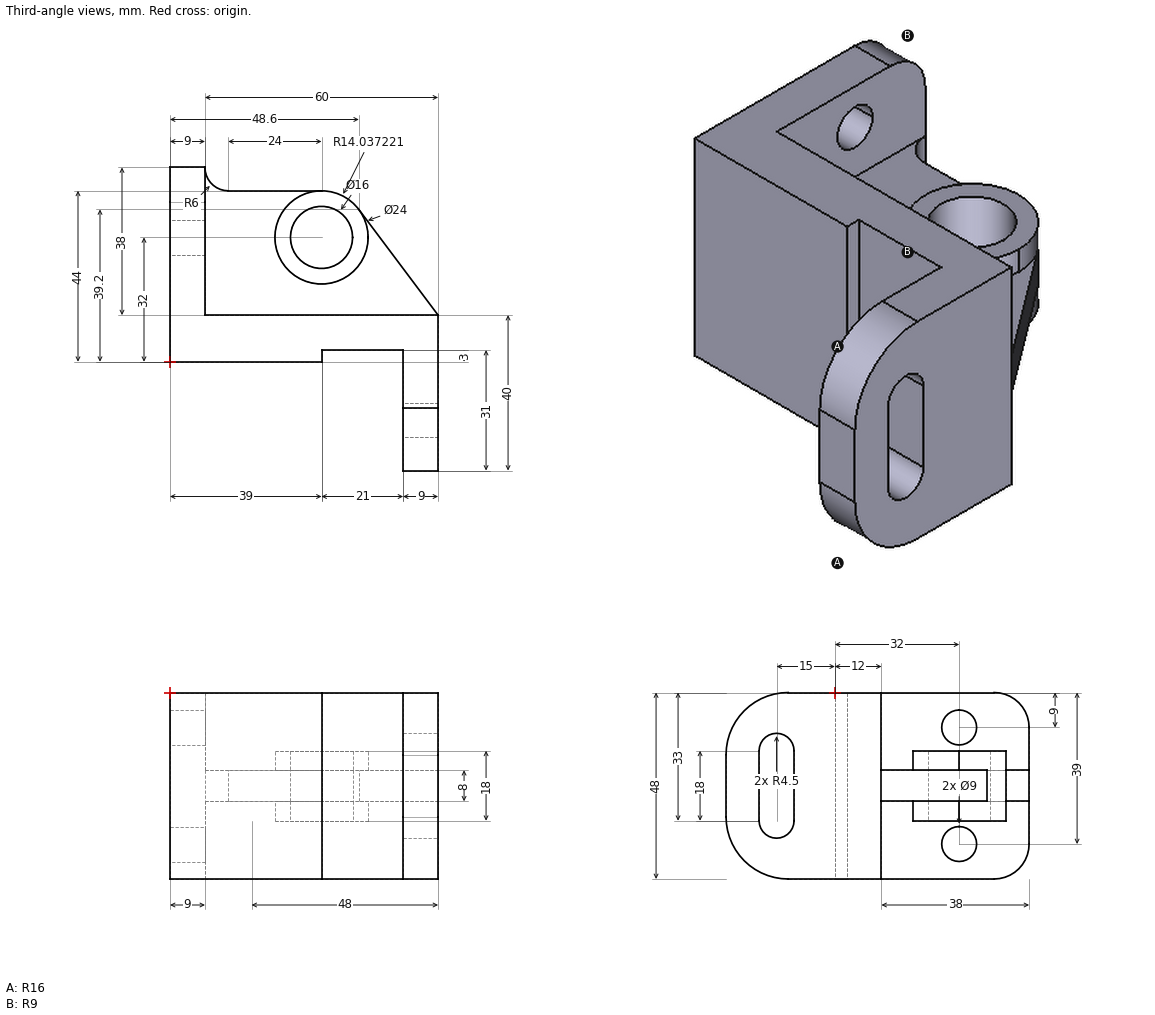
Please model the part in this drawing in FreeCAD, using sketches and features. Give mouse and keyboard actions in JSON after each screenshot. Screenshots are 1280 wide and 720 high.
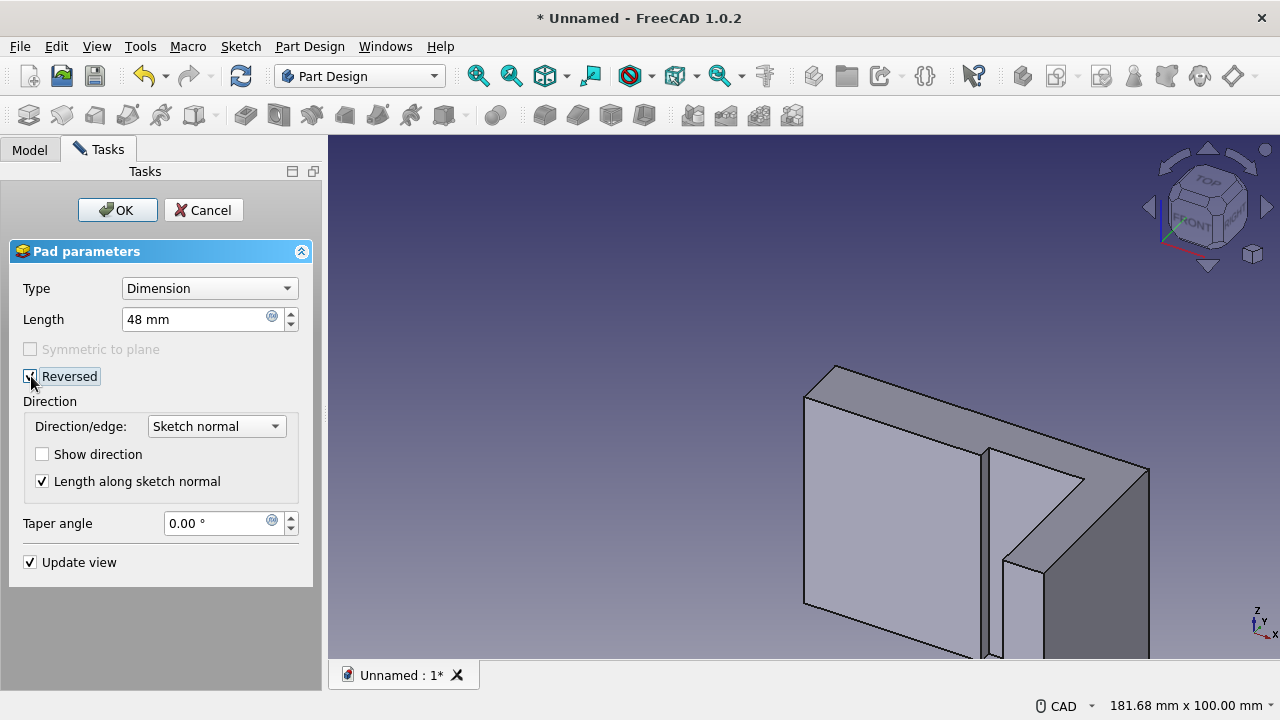
{"action": "left_click", "coordinate": [118, 210]}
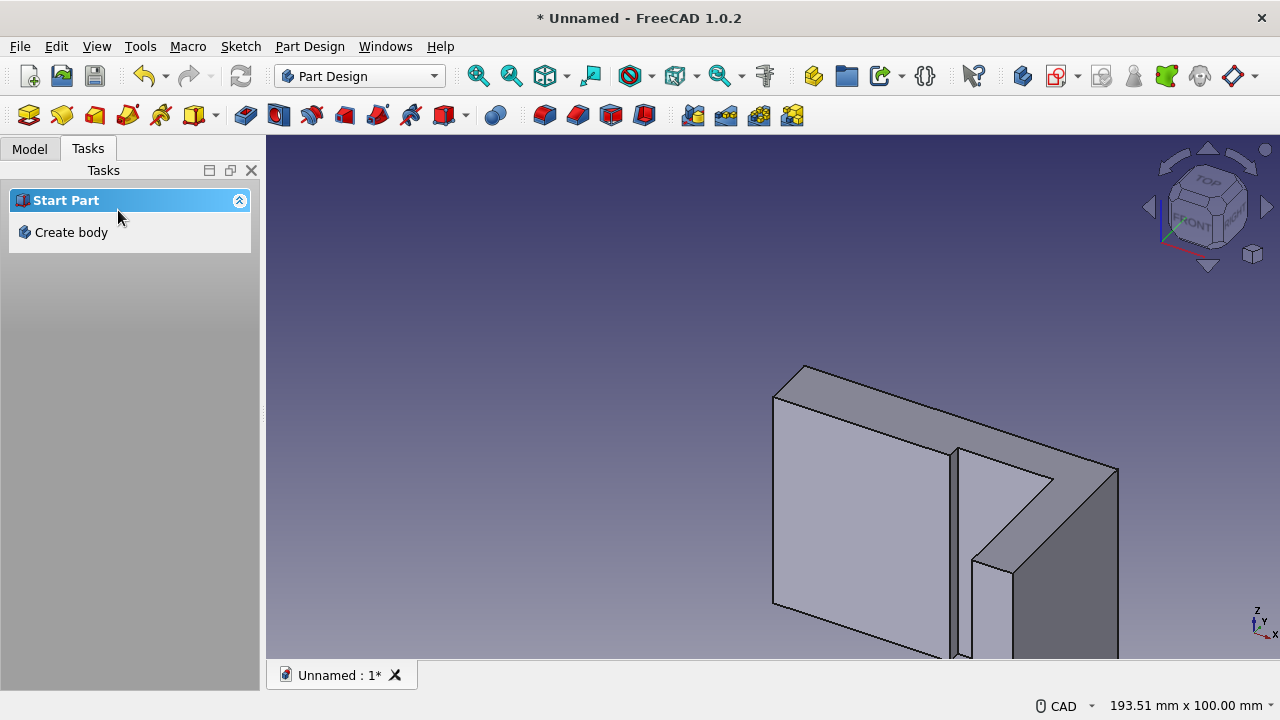
{"action": "key", "text": "v f"}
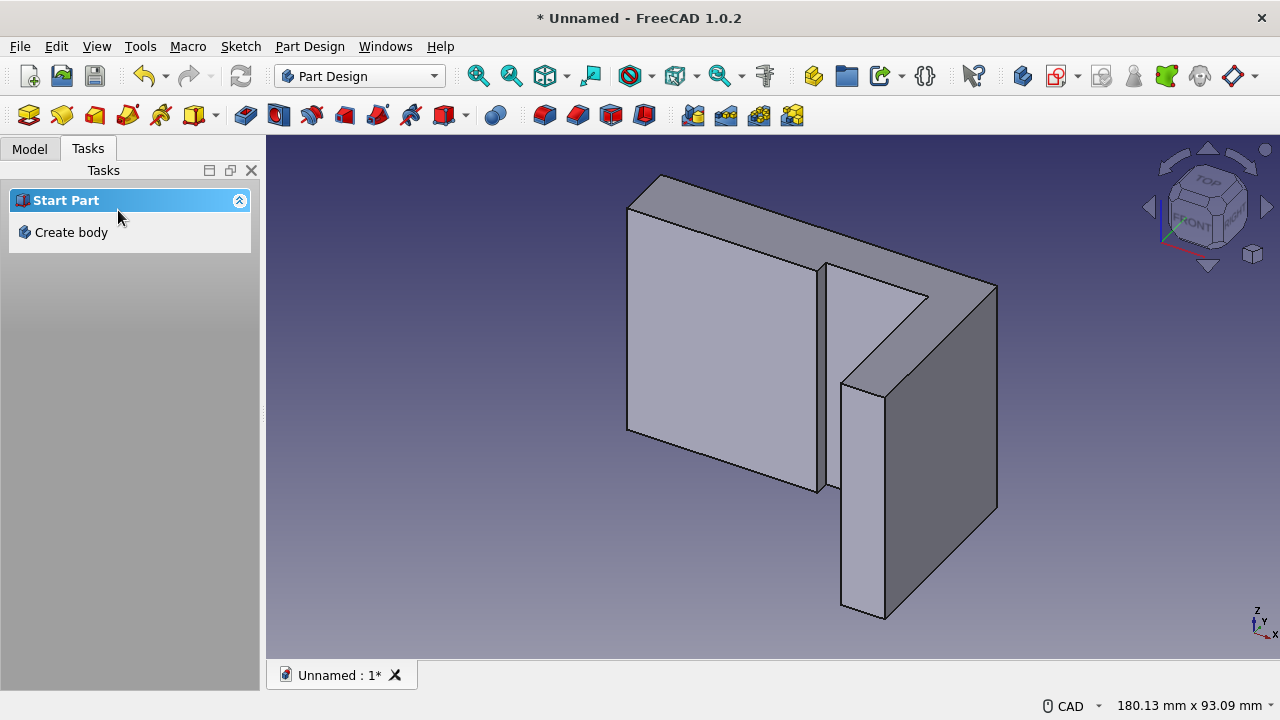
{"action": "left_click", "coordinate": [863, 390]}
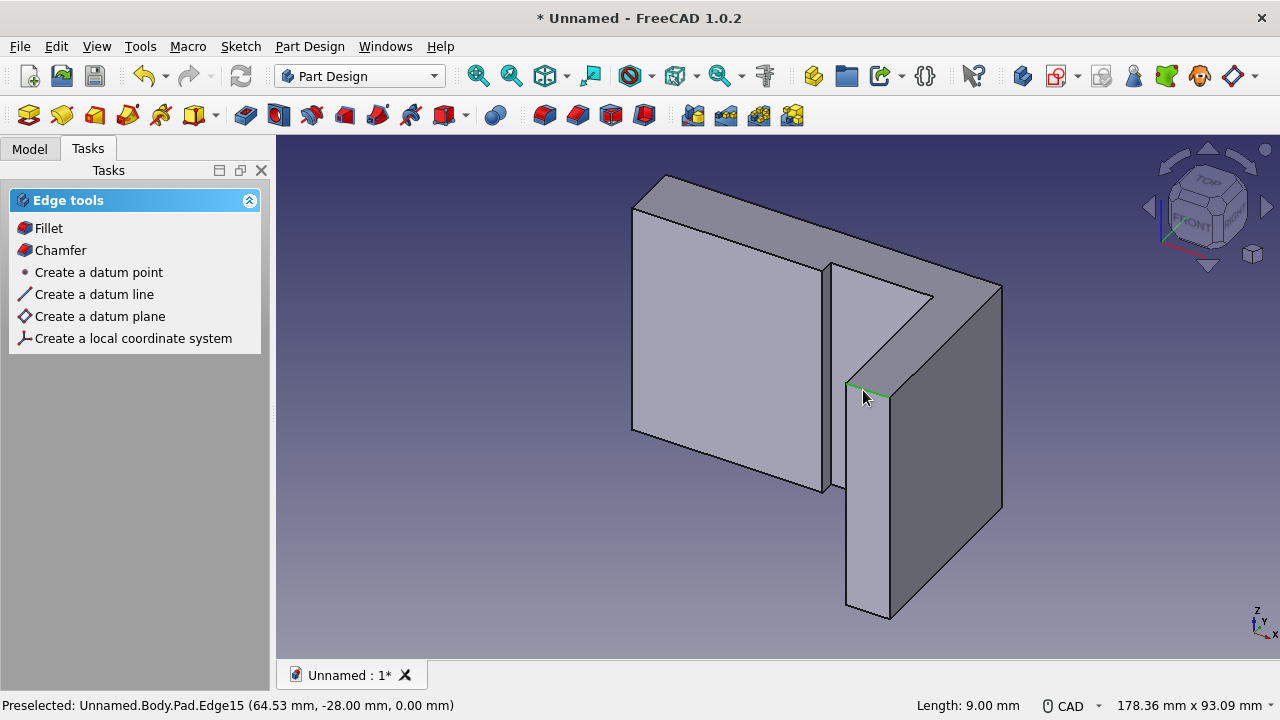
{"action": "key", "text": "0"}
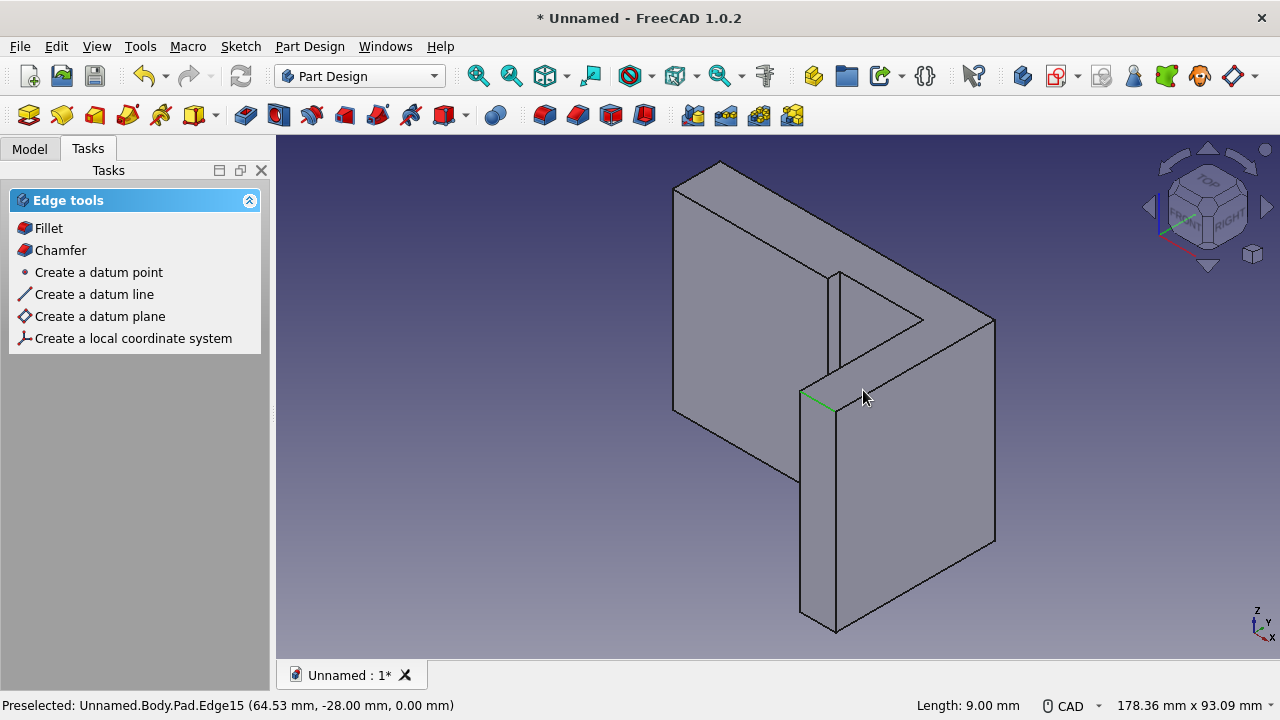
{"action": "key", "text": "2"}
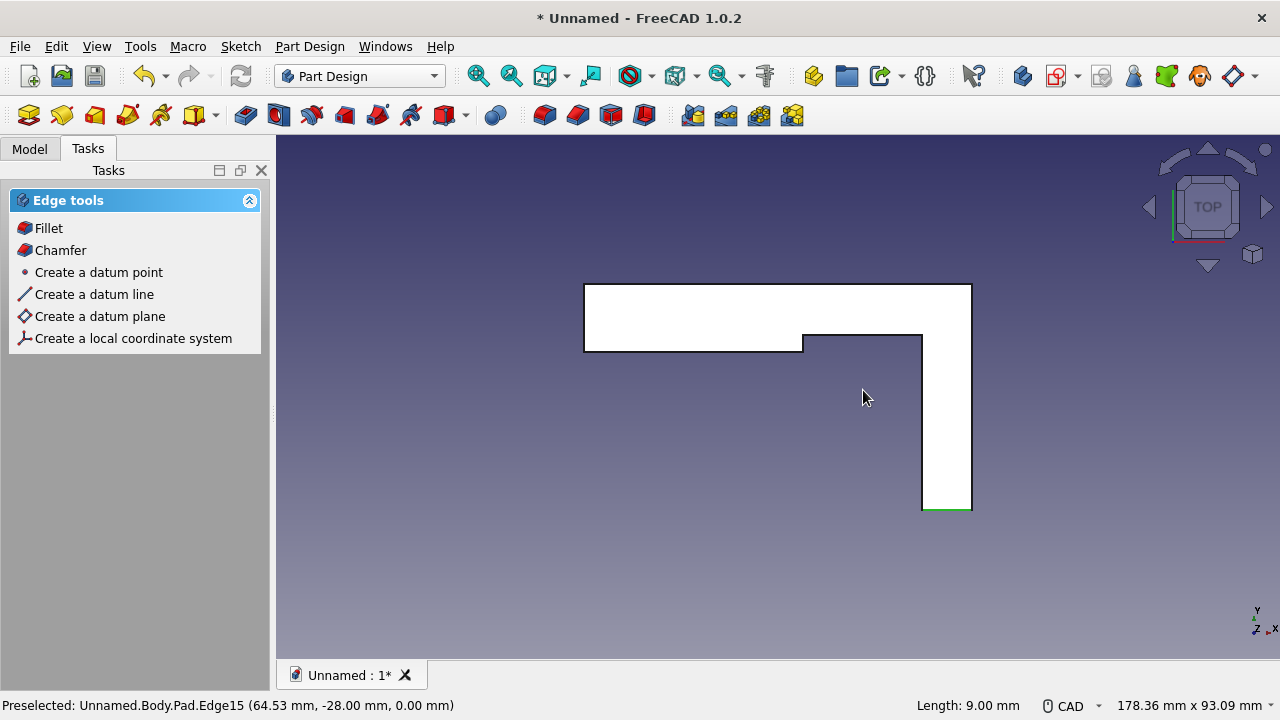
{"action": "key", "text": "v f"}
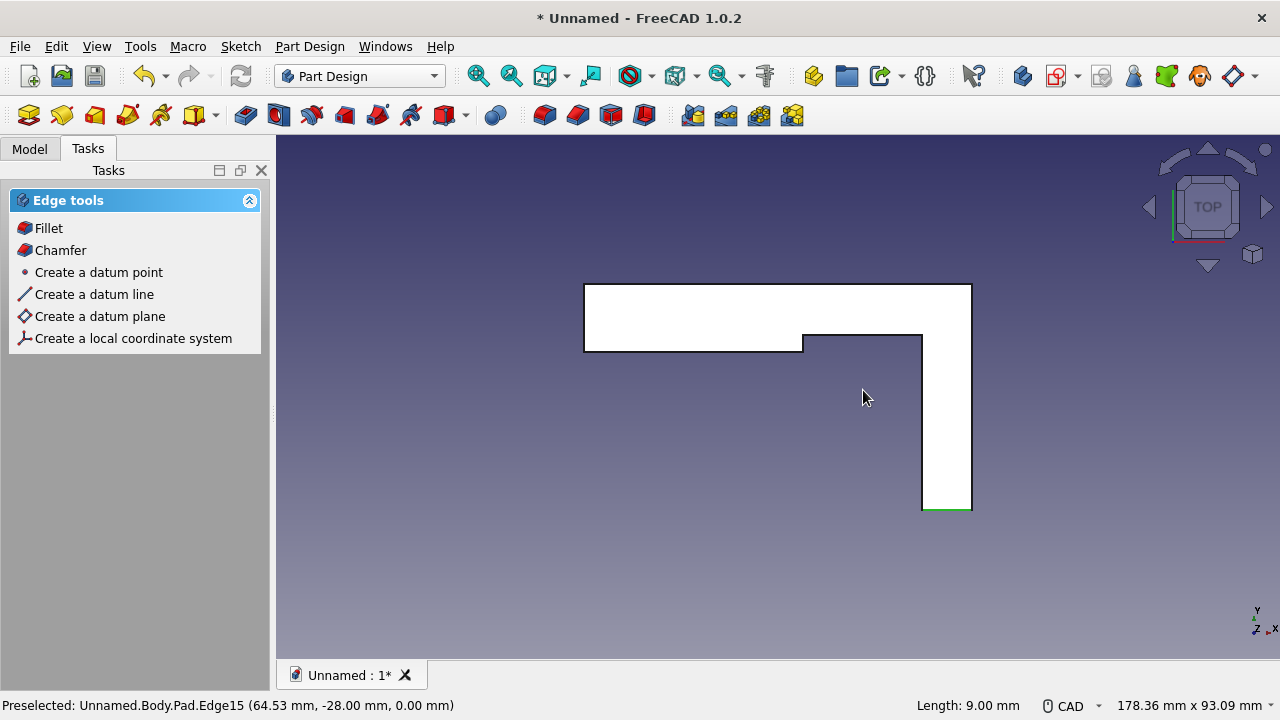
{"action": "key", "text": "1"}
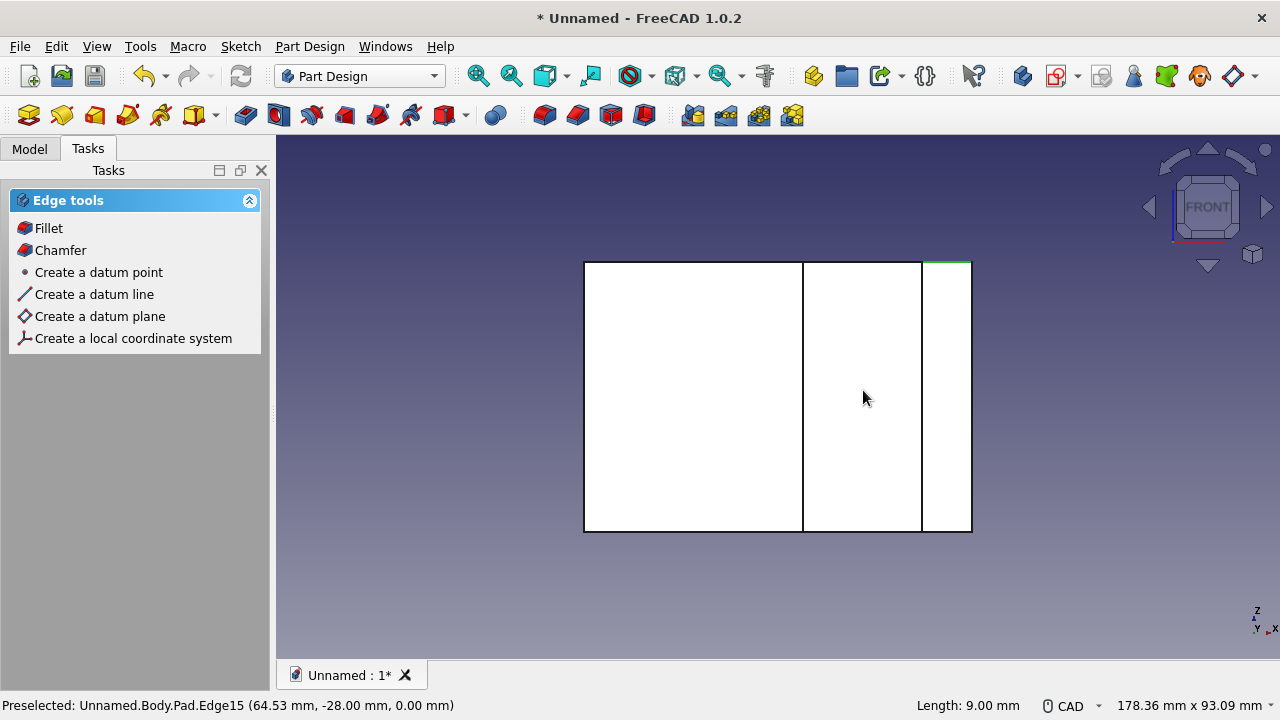
{"action": "left_click", "coordinate": [947, 531], "text": "ctrl"}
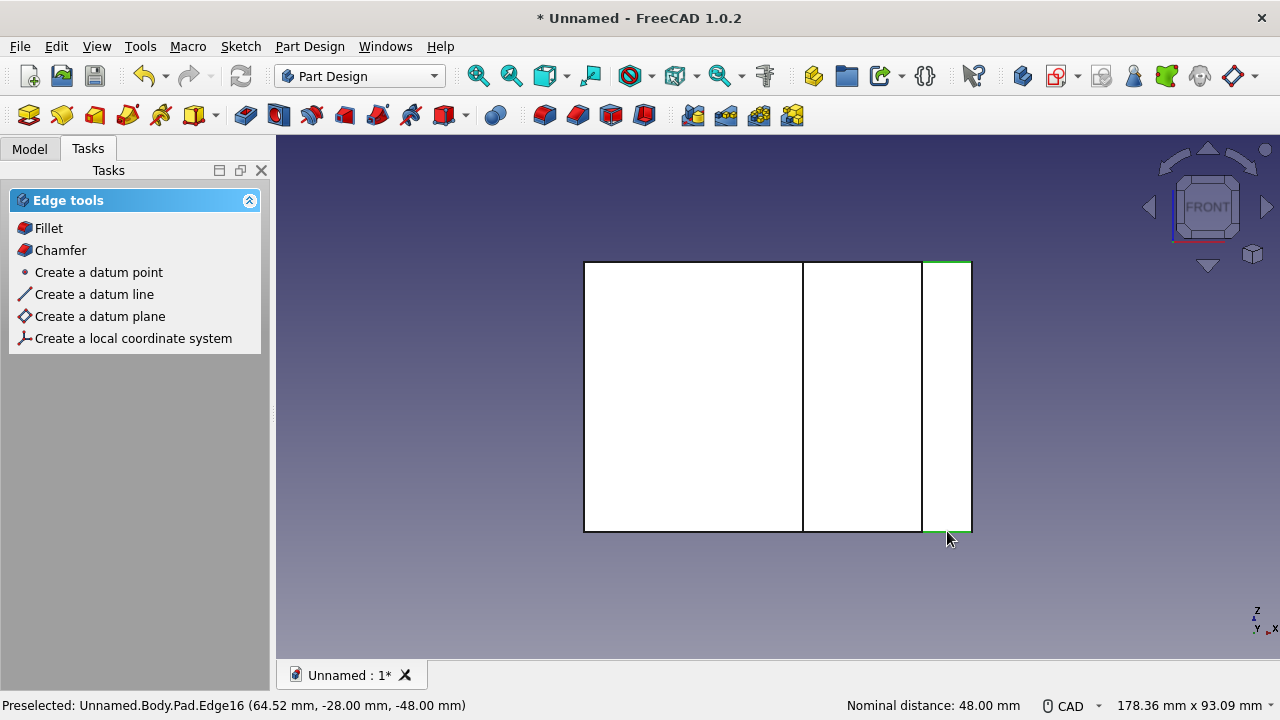
{"action": "left_click", "coordinate": [545, 116]}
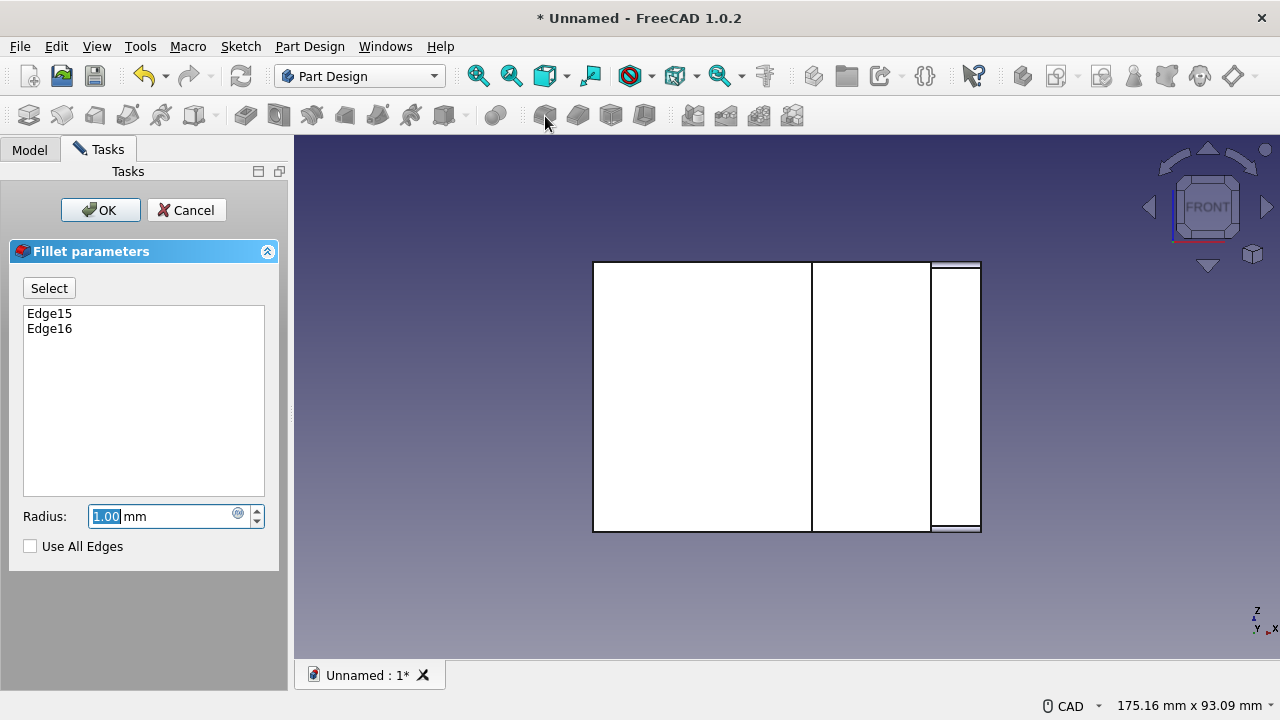
{"action": "type", "text": "16"}
{"action": "key", "text": "Tab"}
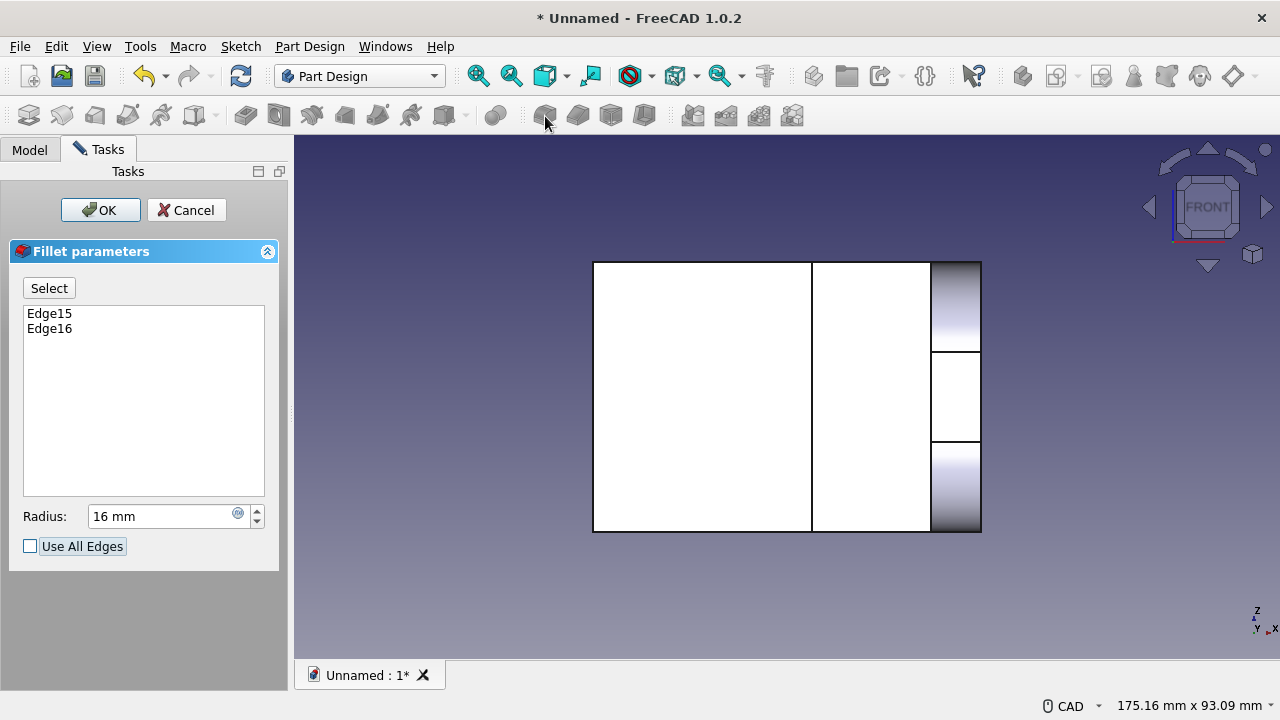
{"action": "left_click", "coordinate": [101, 210]}